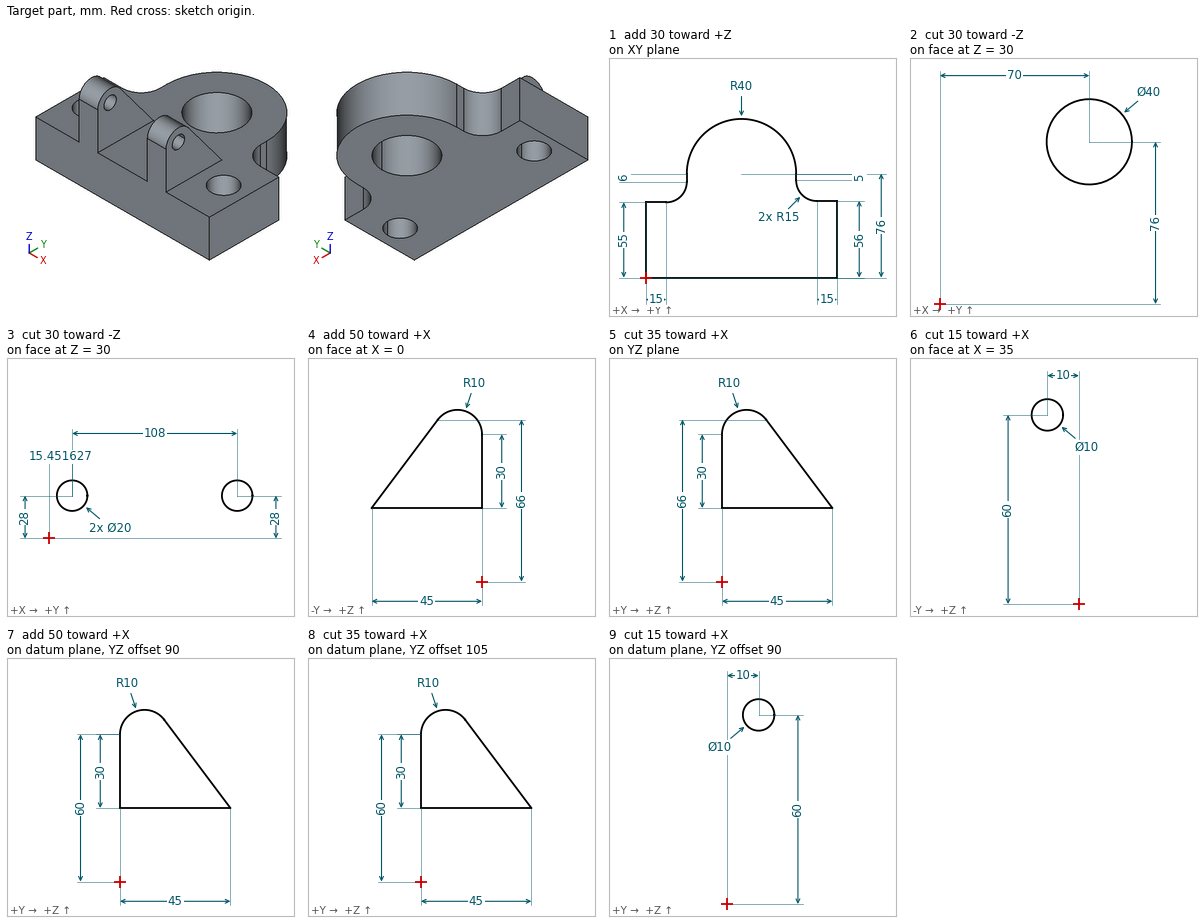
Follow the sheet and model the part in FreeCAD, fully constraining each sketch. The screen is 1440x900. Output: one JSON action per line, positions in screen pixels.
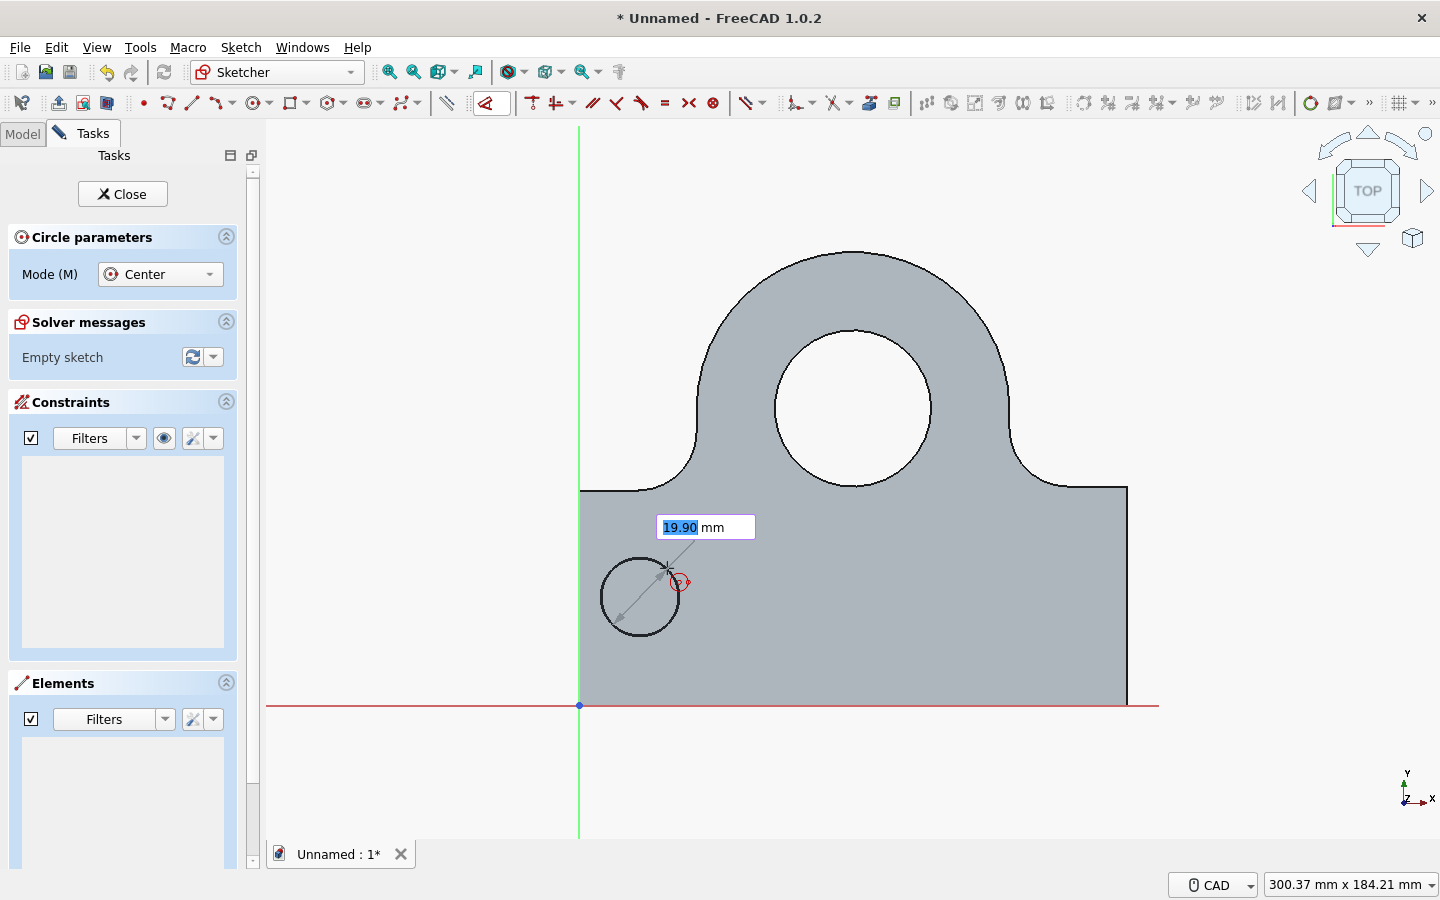
{"action": "type", "text": "20"}
{"action": "key", "text": "Return"}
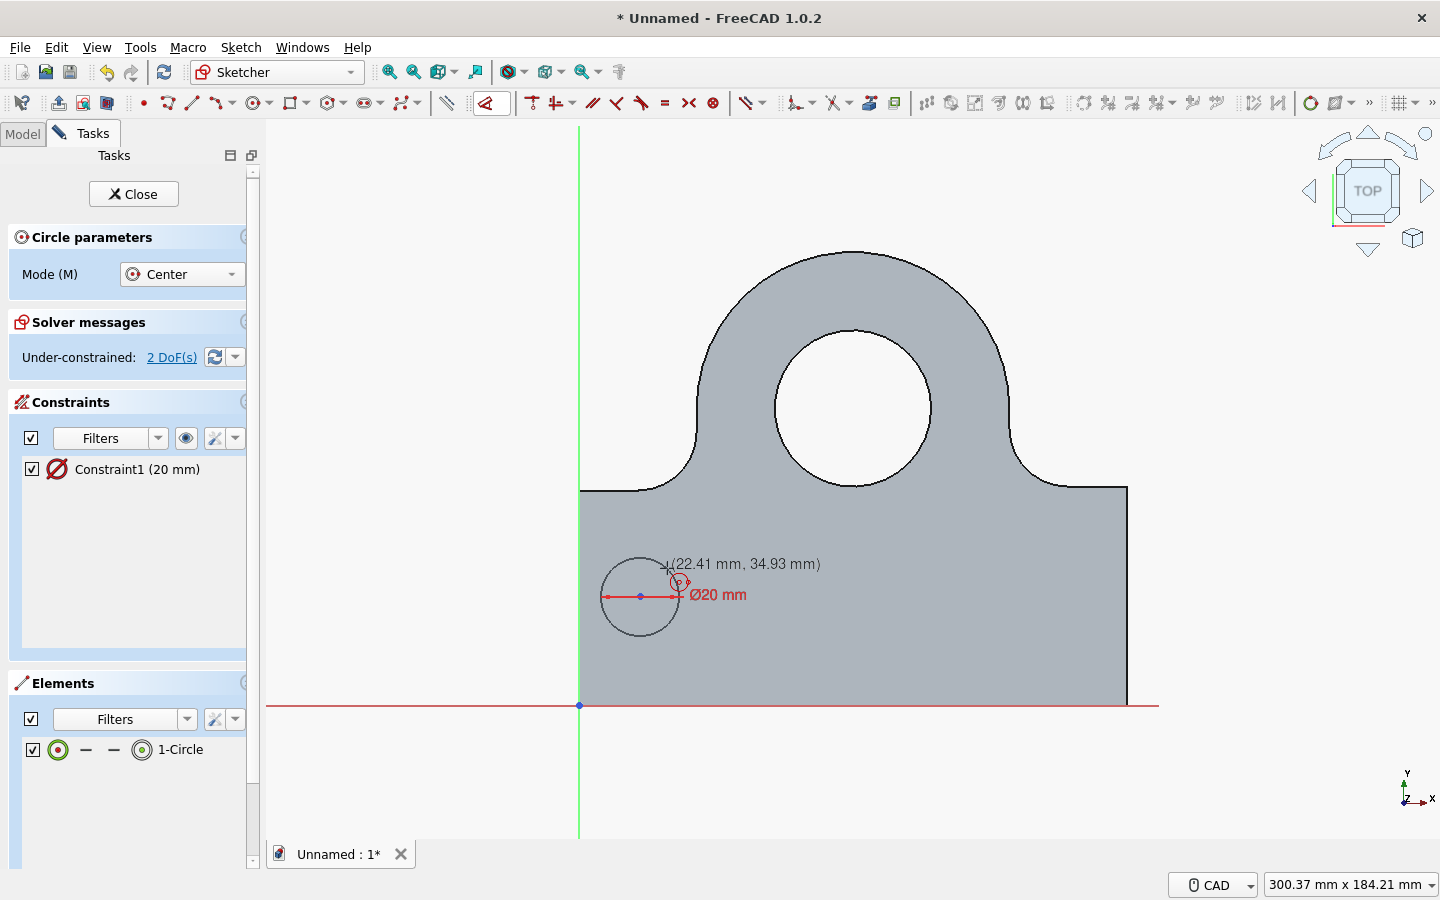
{"action": "left_click", "coordinate": [1062, 596]}
{"action": "mouse_move", "coordinate": [1090, 568]}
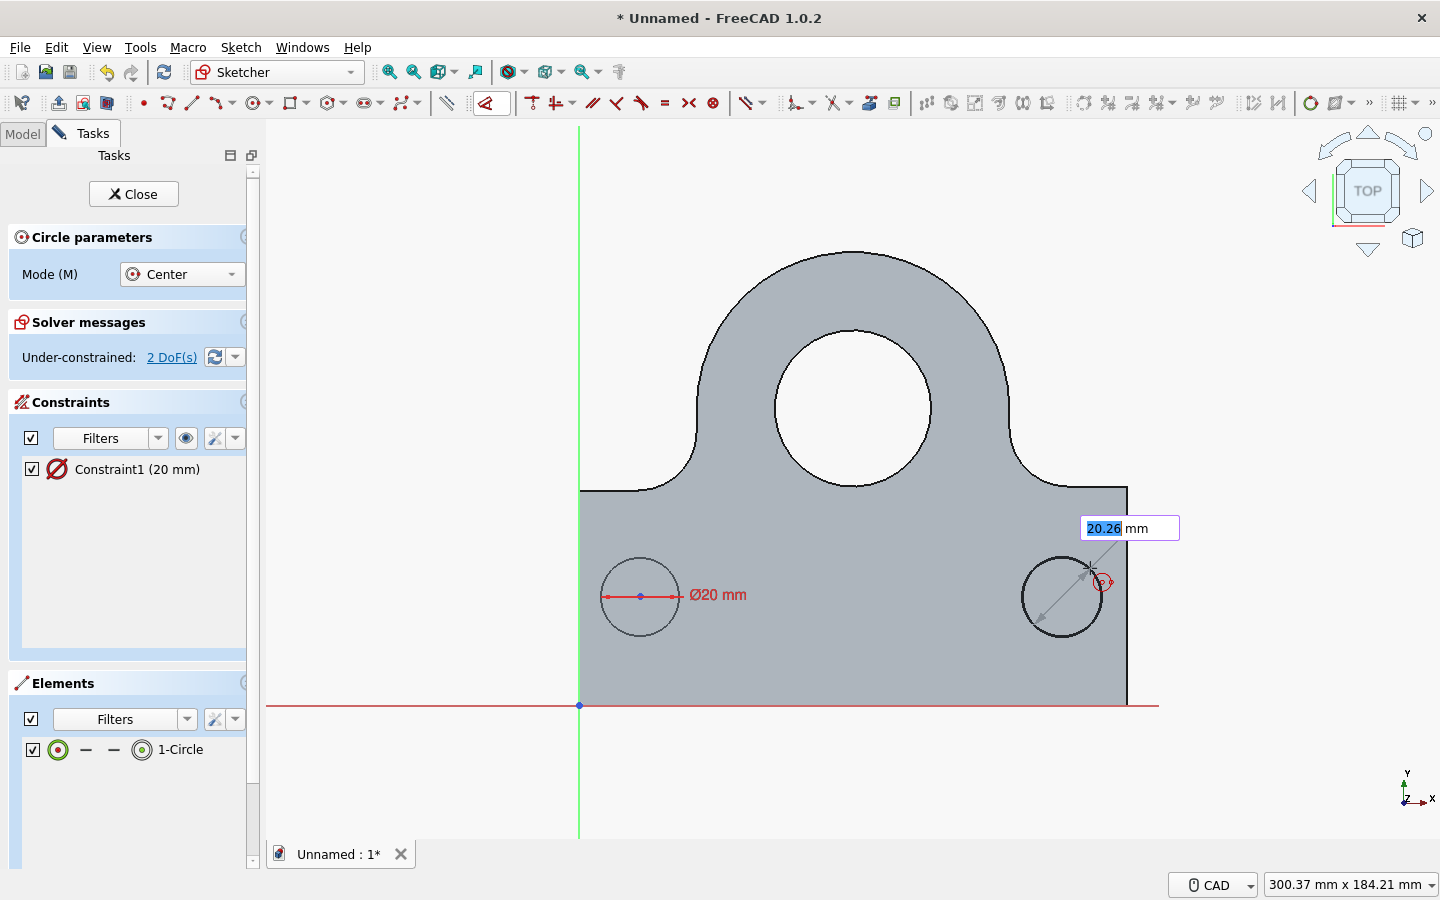
{"action": "type", "text": "20"}
{"action": "key", "text": "Return"}
{"action": "key", "text": "Escape"}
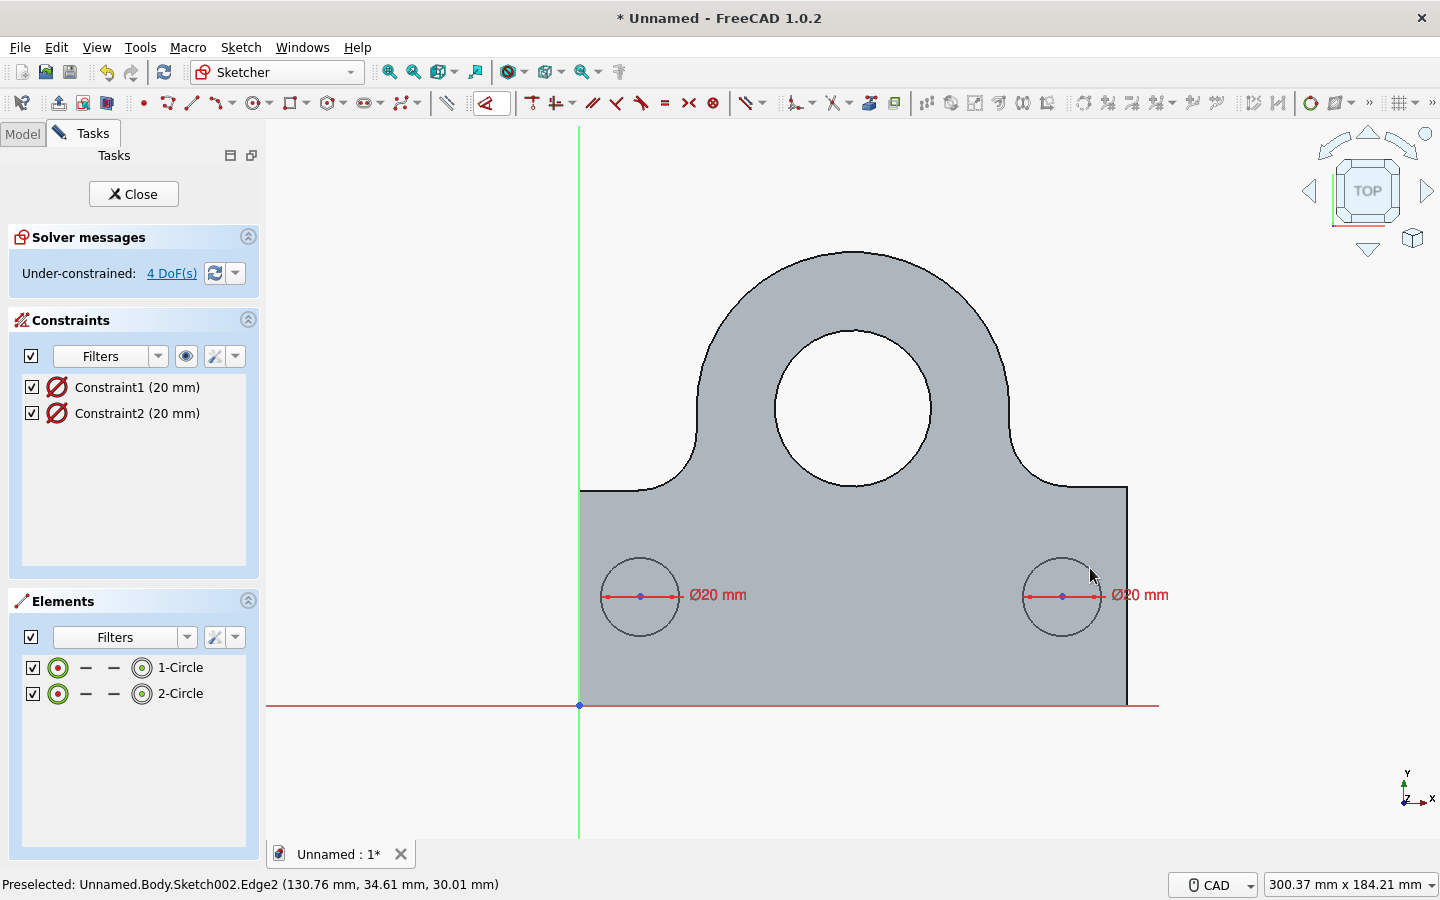
{"action": "left_click", "coordinate": [640, 597]}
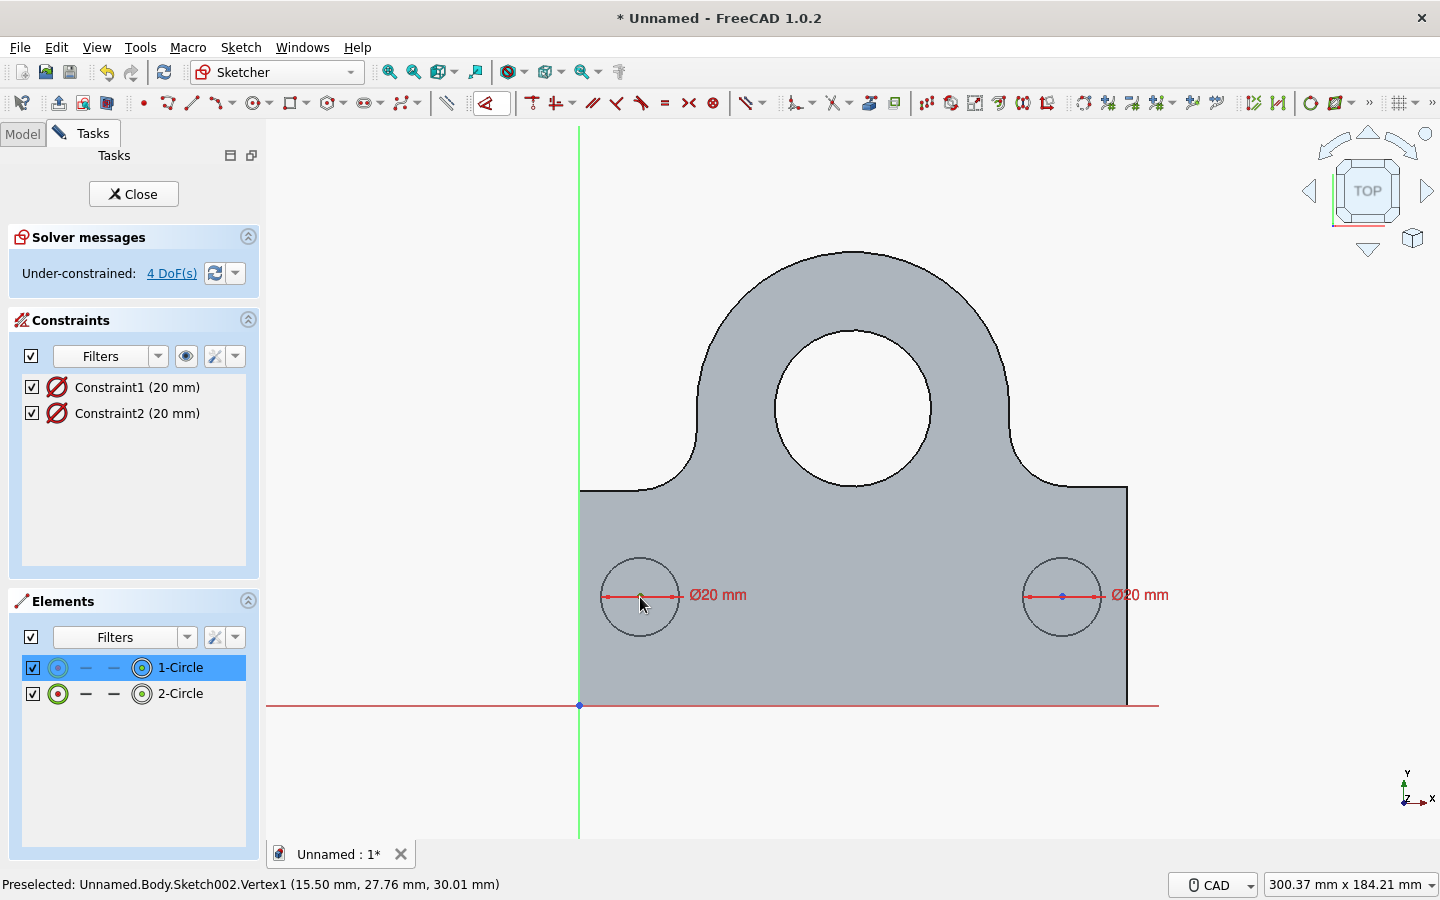
{"action": "key", "text": "i"}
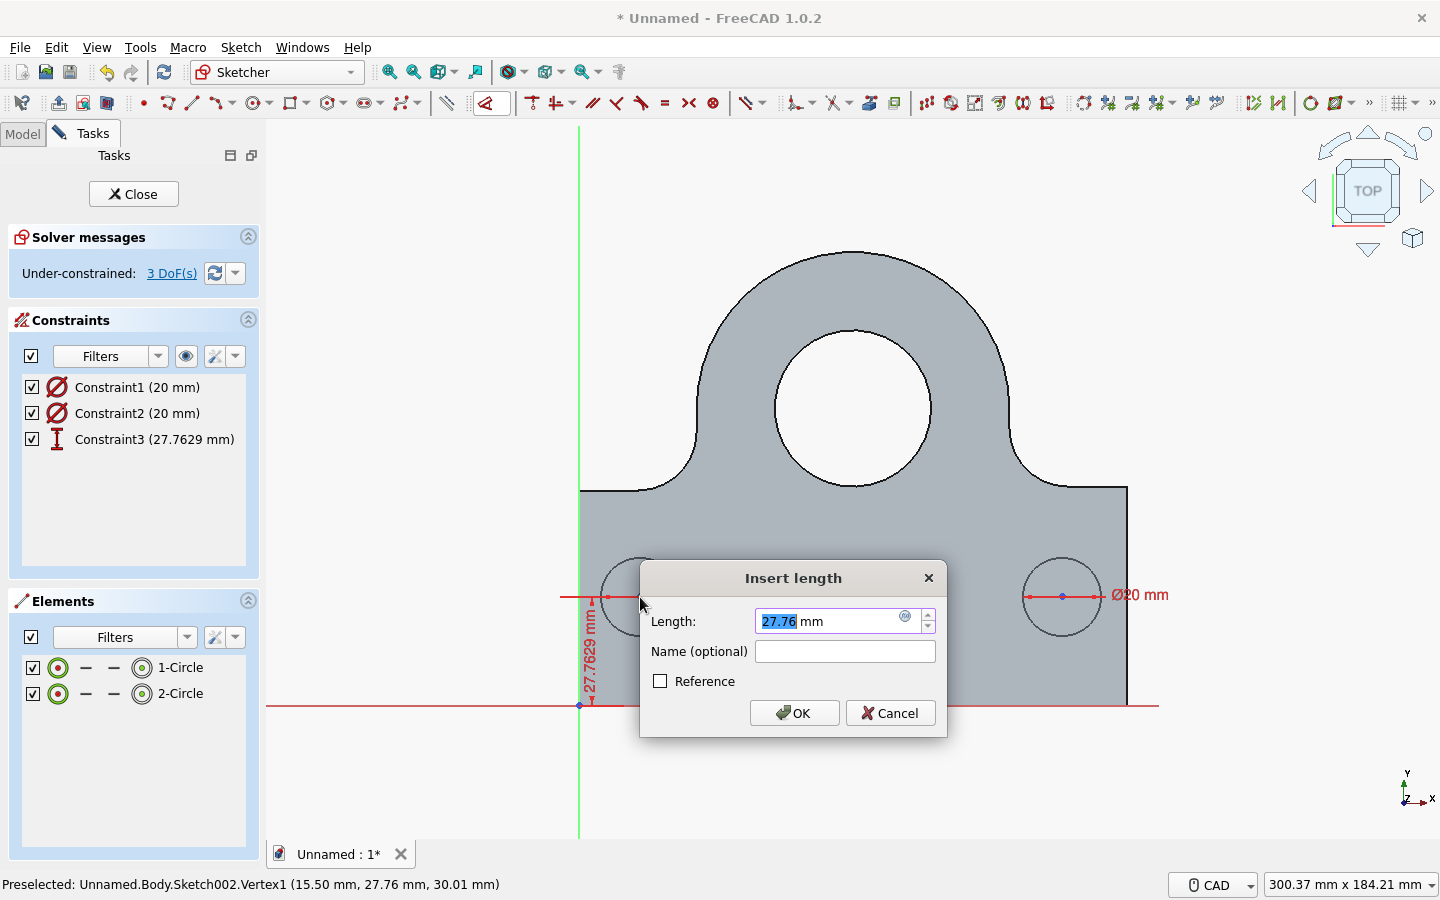
{"action": "type", "text": "28"}
{"action": "key", "text": "Return"}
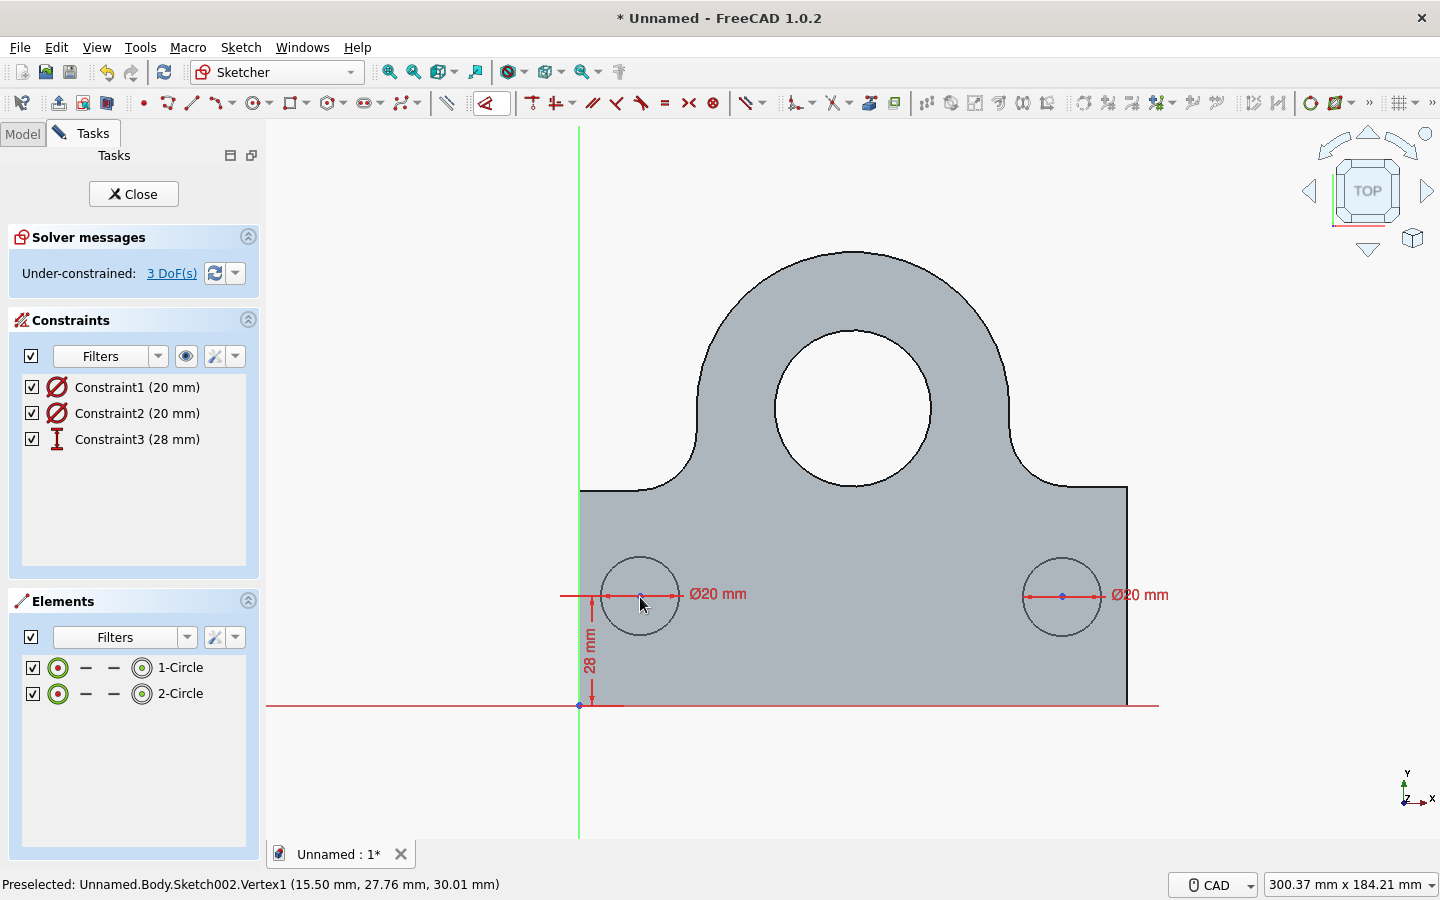
{"action": "left_click", "coordinate": [1062, 597]}